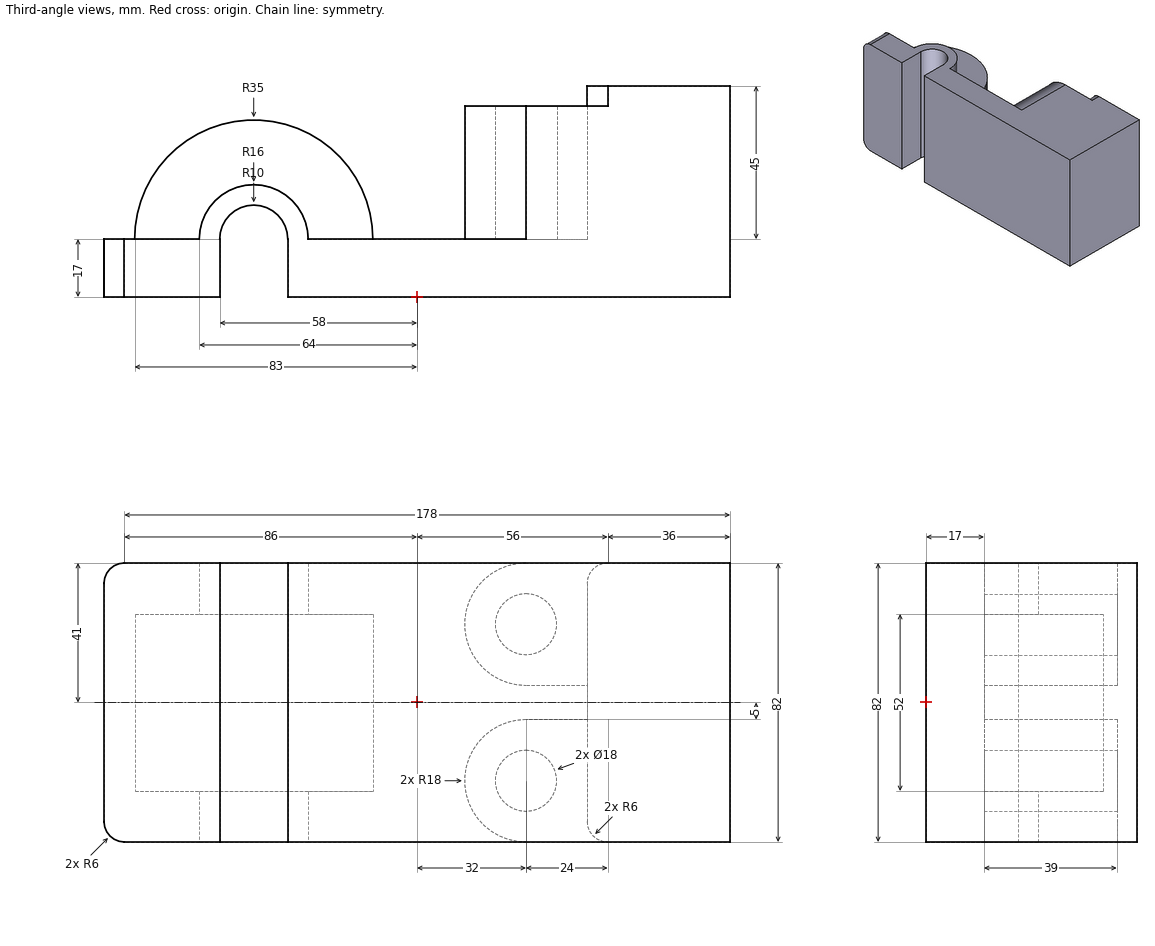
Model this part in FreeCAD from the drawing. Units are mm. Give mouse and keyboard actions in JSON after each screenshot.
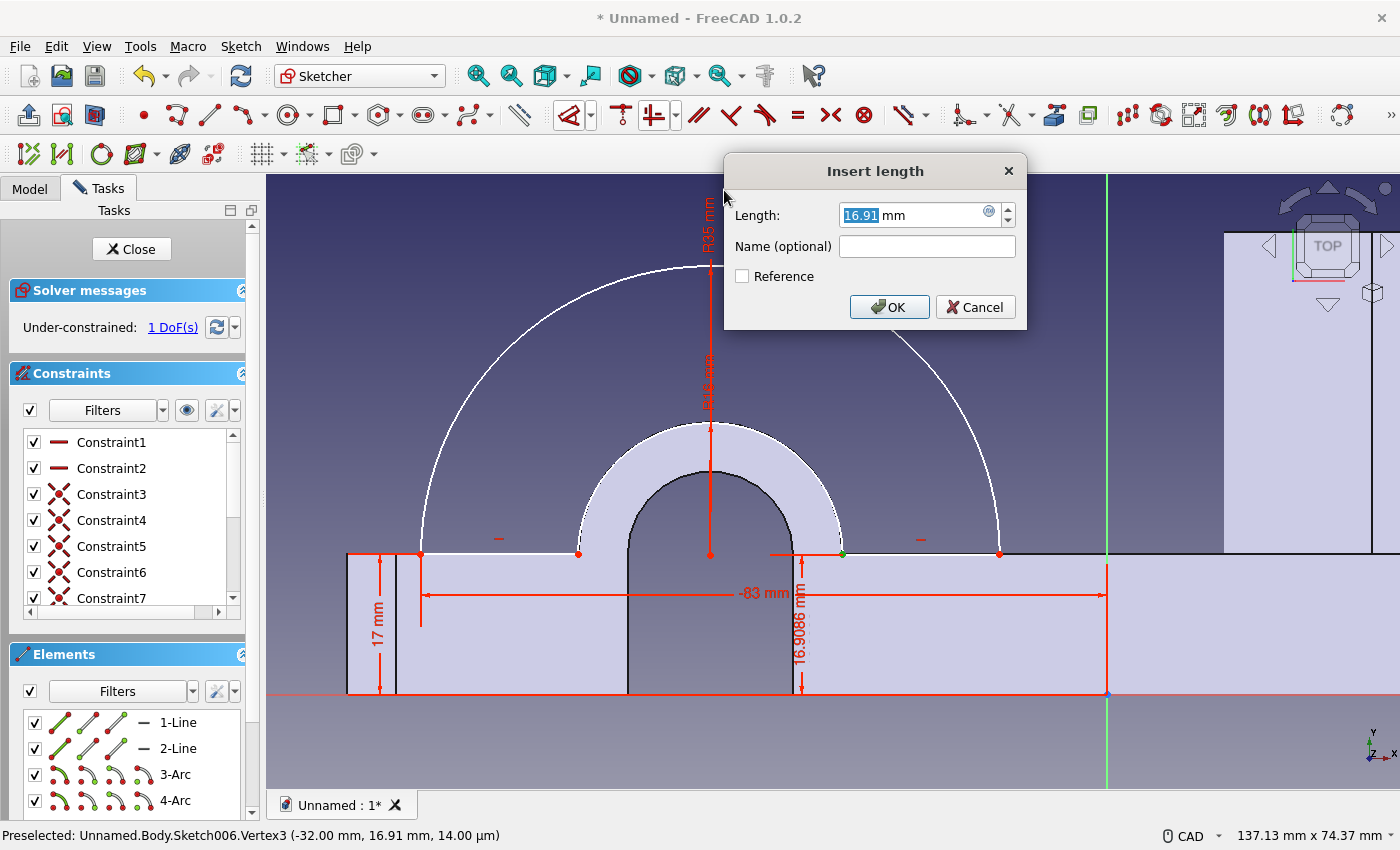
{"action": "type", "text": "17"}
{"action": "key", "text": "Return"}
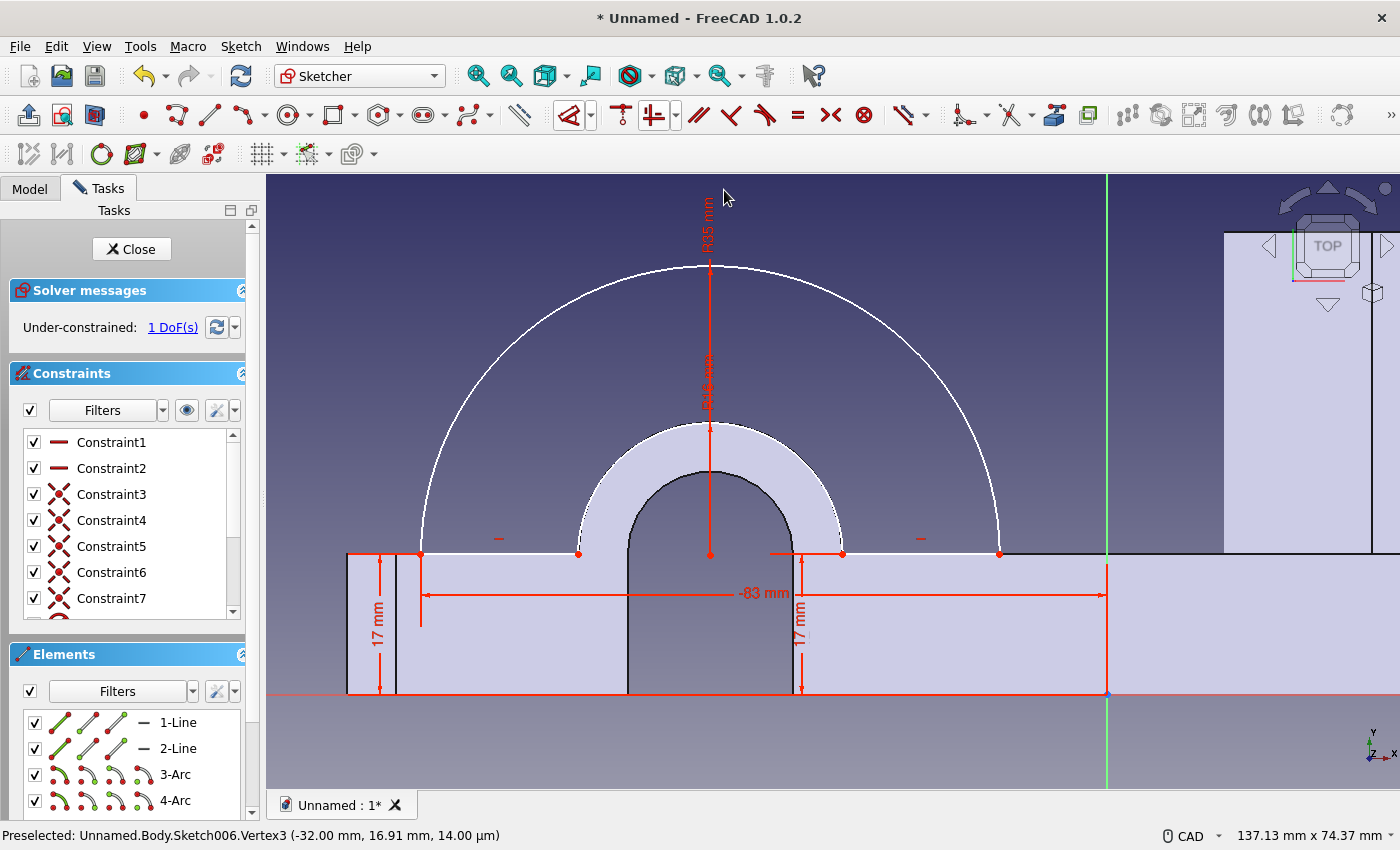
{"action": "left_click", "coordinate": [710, 556]}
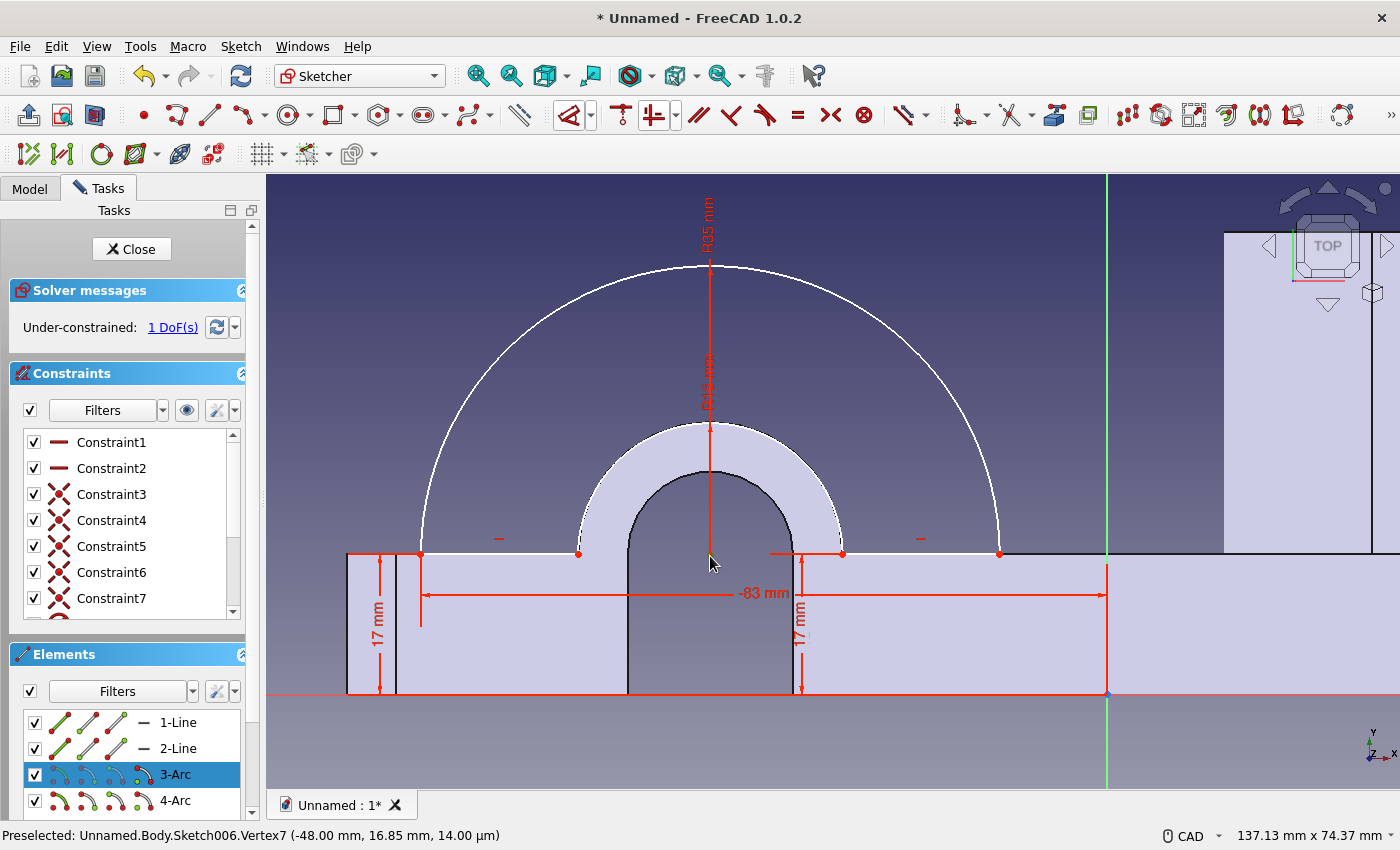
{"action": "left_click", "coordinate": [590, 116]}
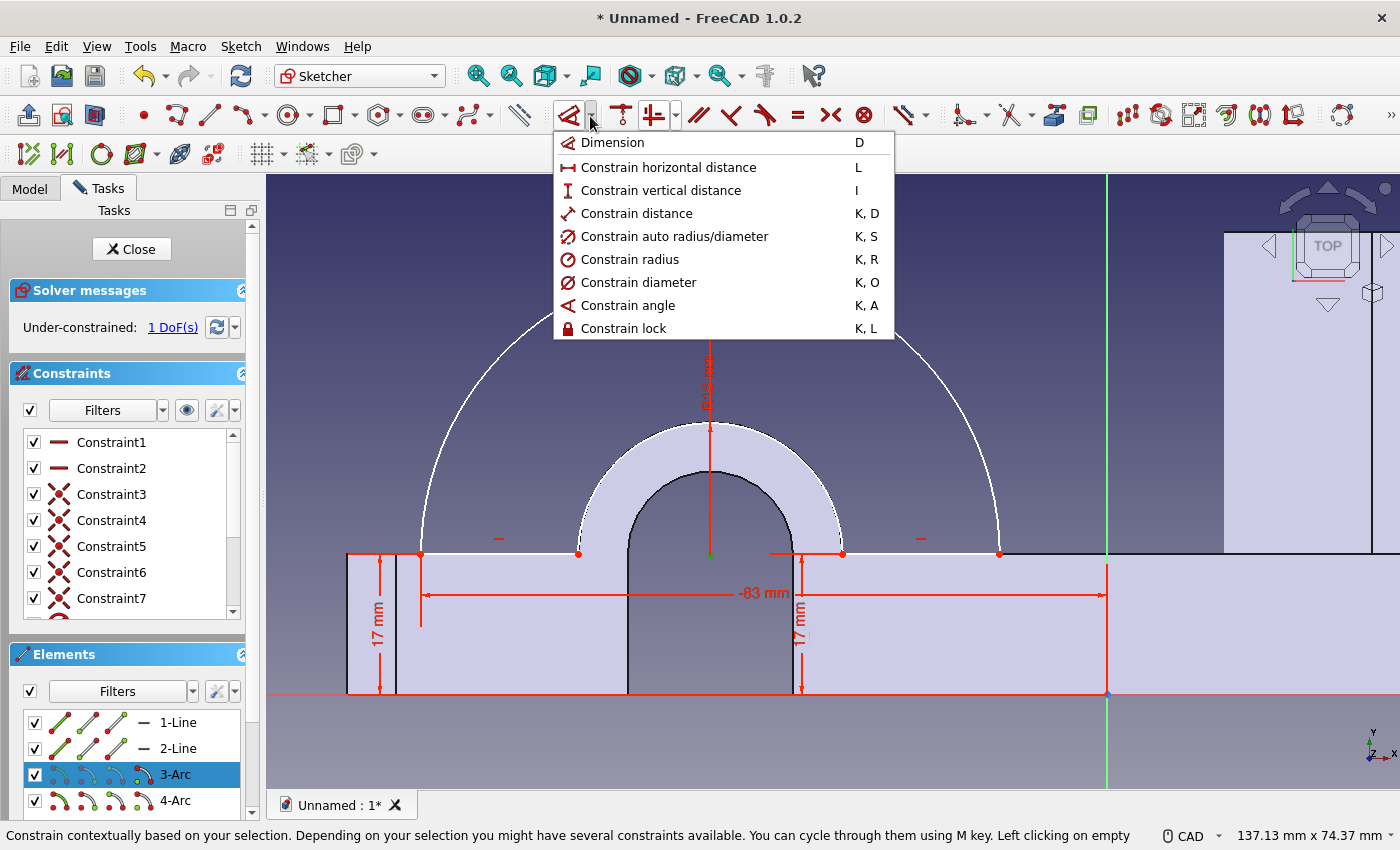
{"action": "left_click", "coordinate": [724, 190]}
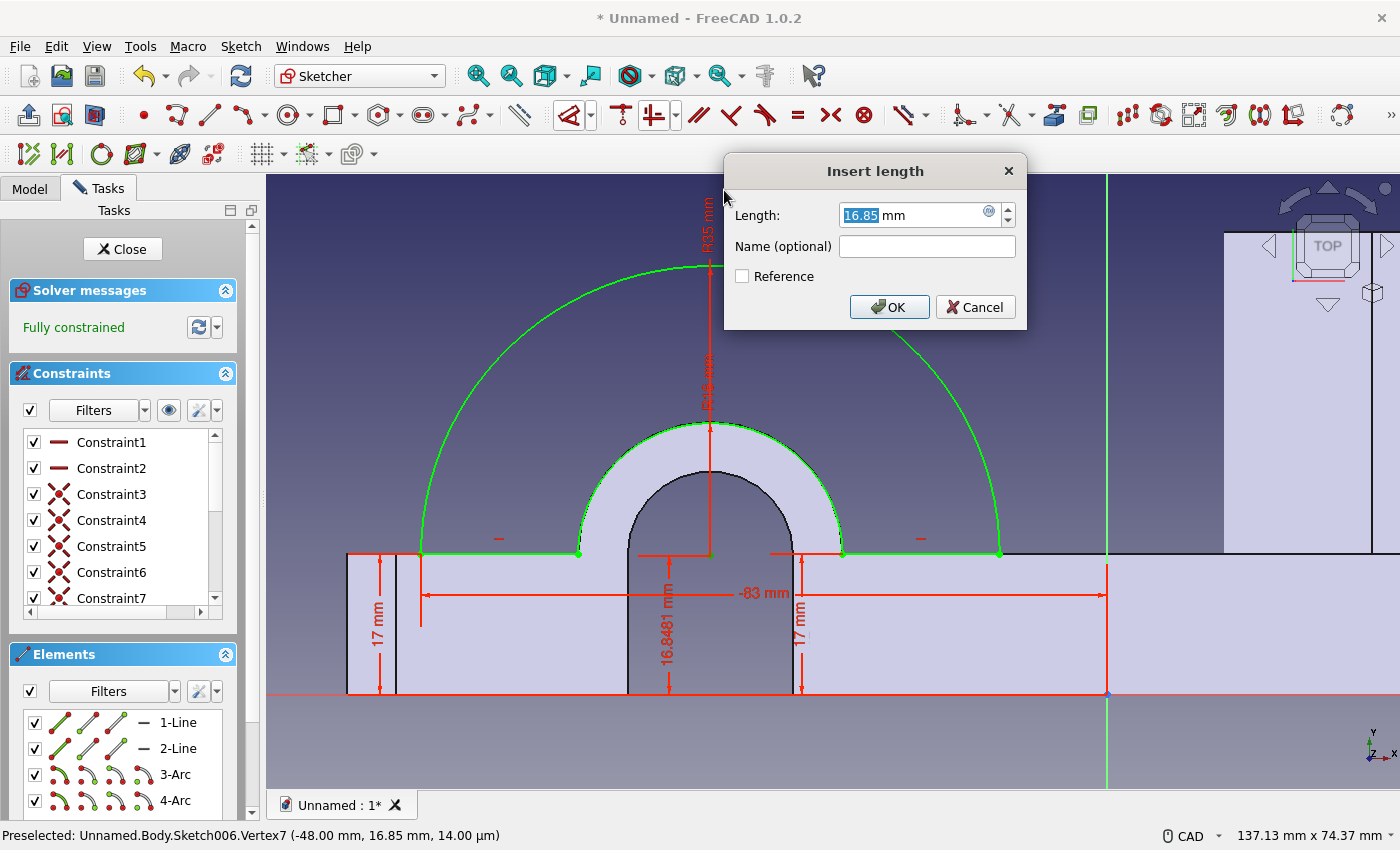
{"action": "type", "text": "17"}
{"action": "key", "text": "Return"}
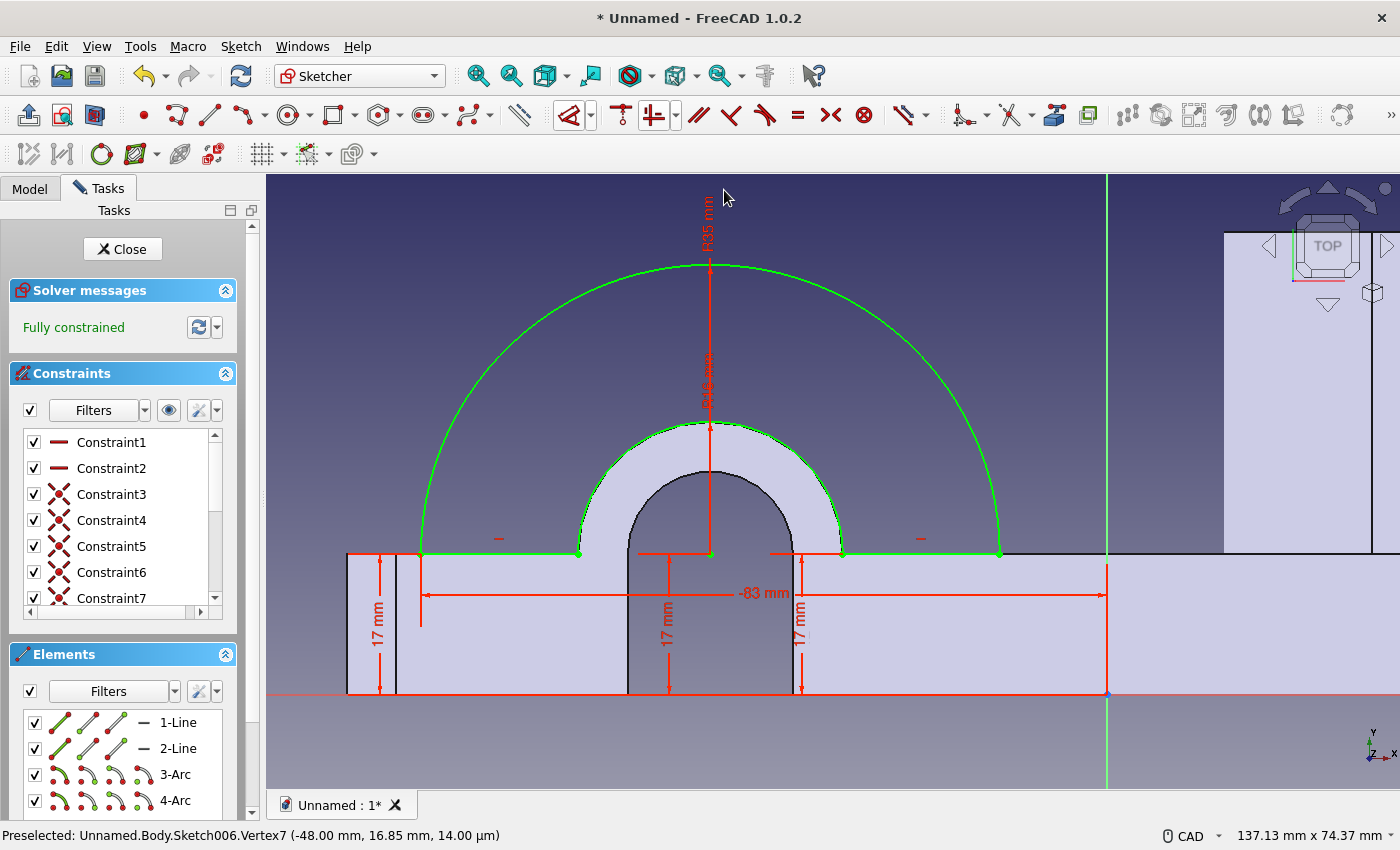
{"action": "left_click", "coordinate": [123, 249]}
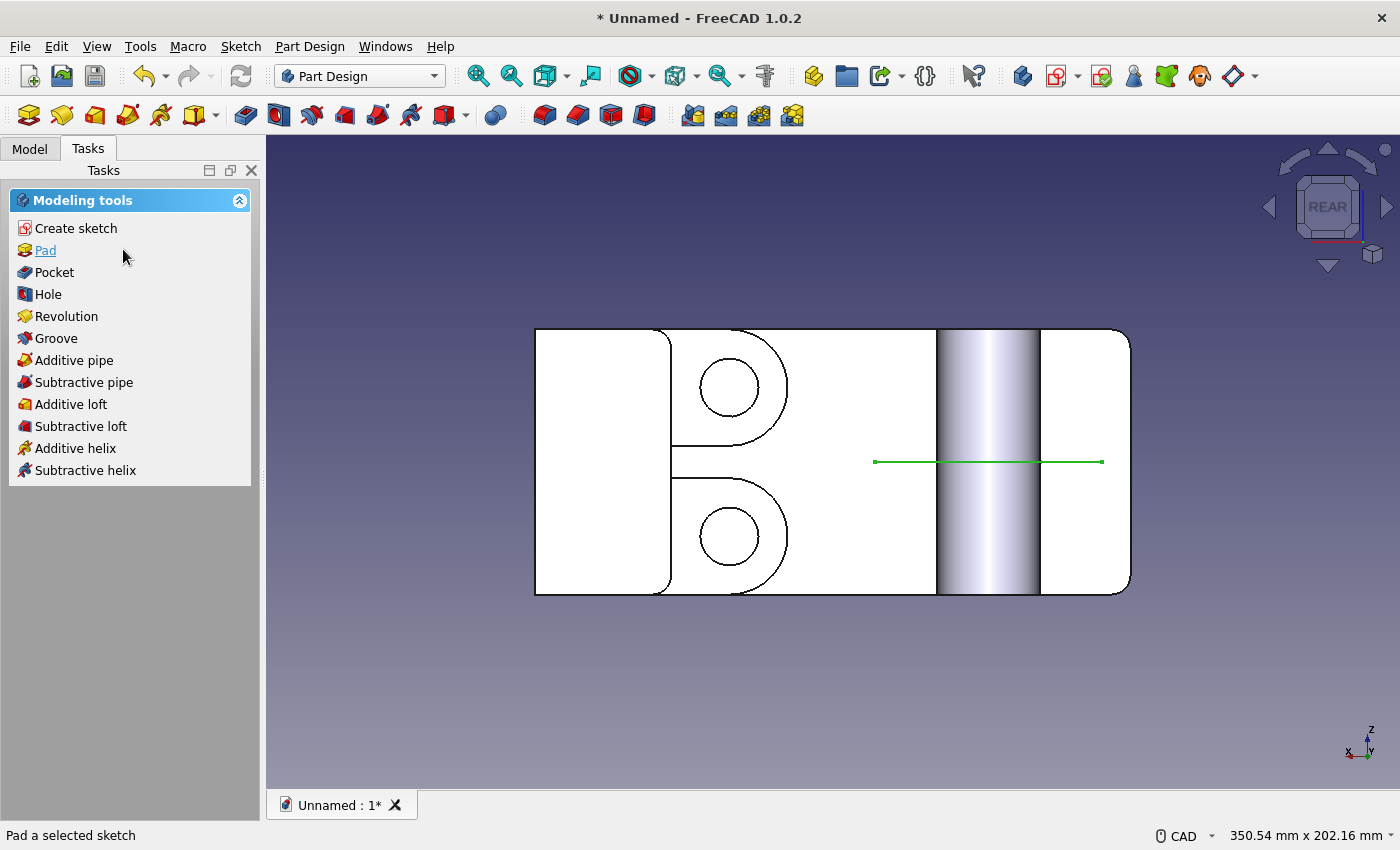
{"action": "left_click", "coordinate": [29, 116]}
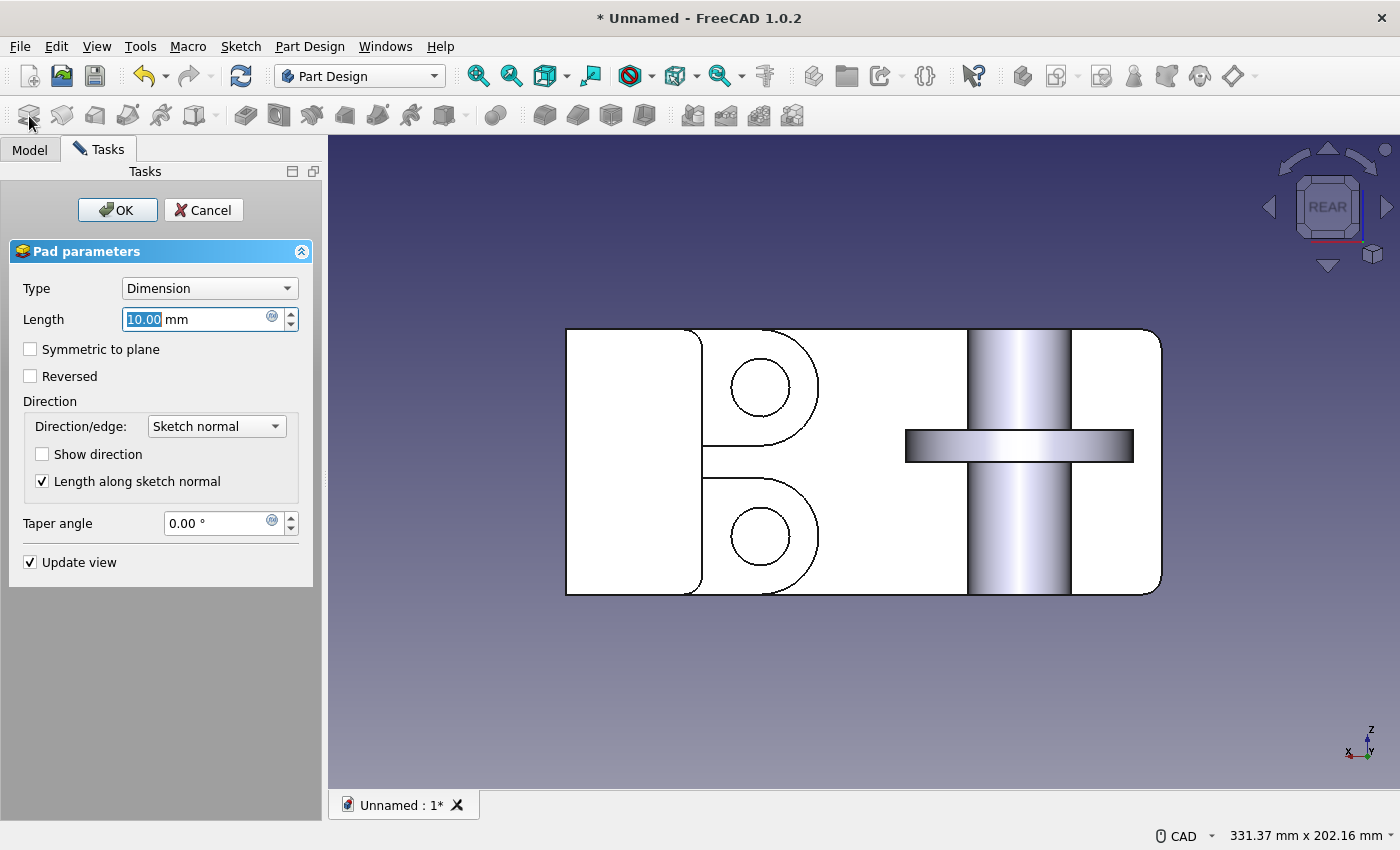
{"action": "type", "text": "52"}
{"action": "key", "text": "Tab"}